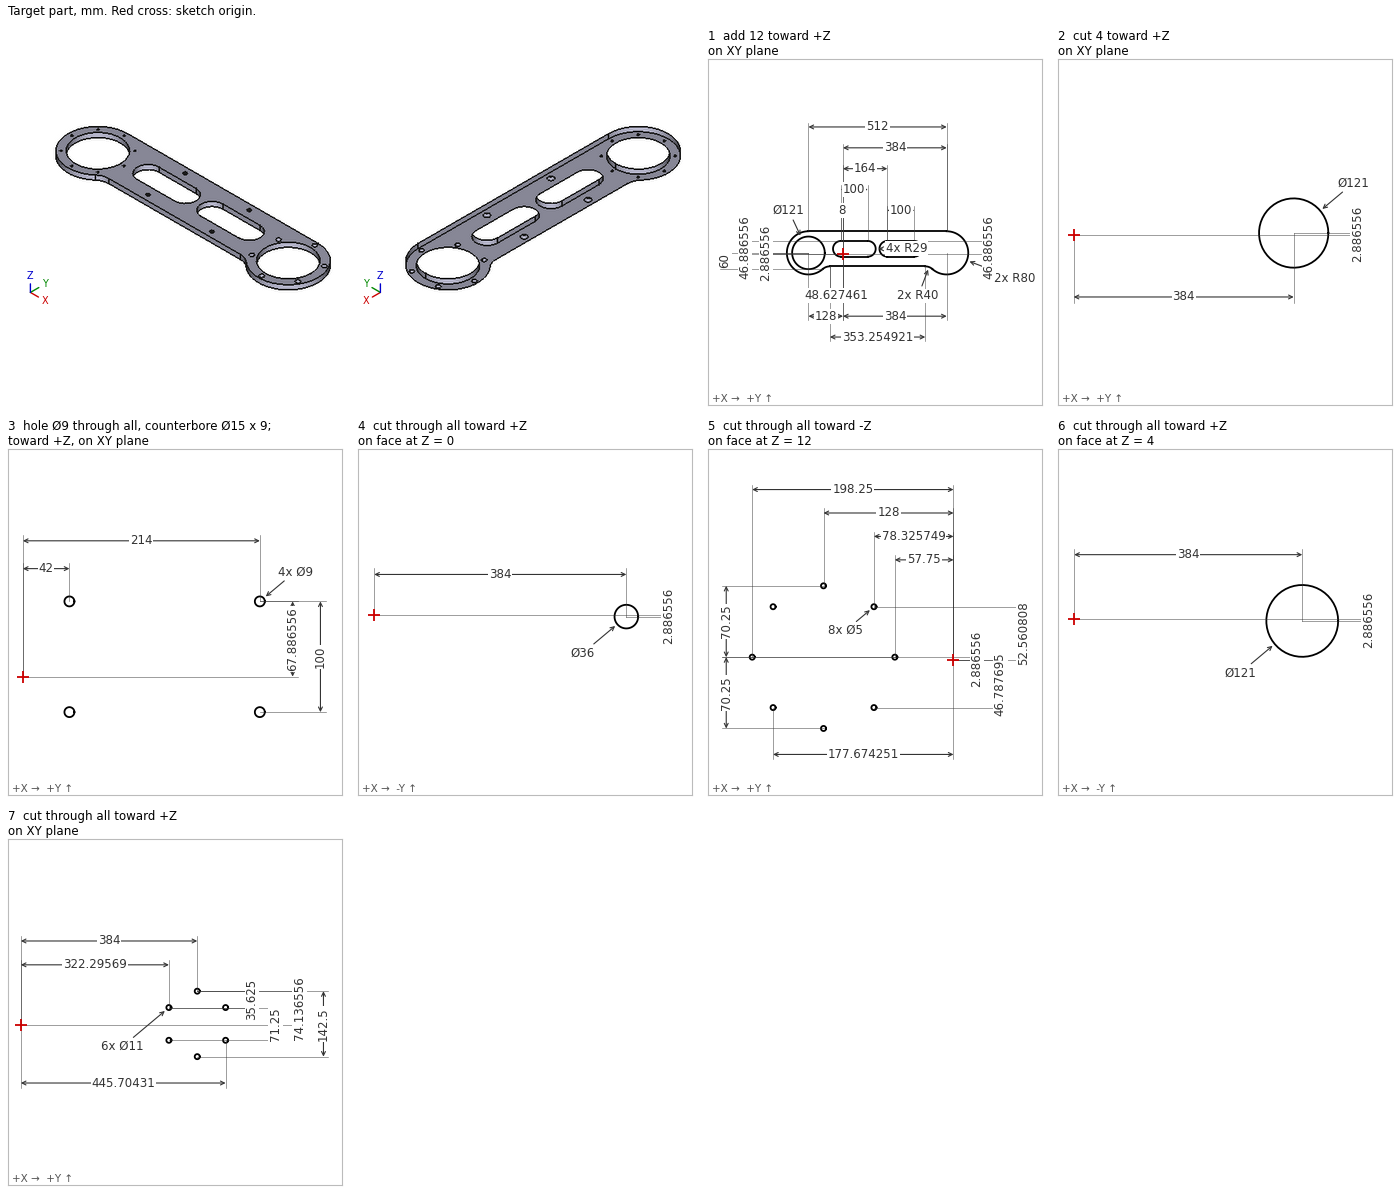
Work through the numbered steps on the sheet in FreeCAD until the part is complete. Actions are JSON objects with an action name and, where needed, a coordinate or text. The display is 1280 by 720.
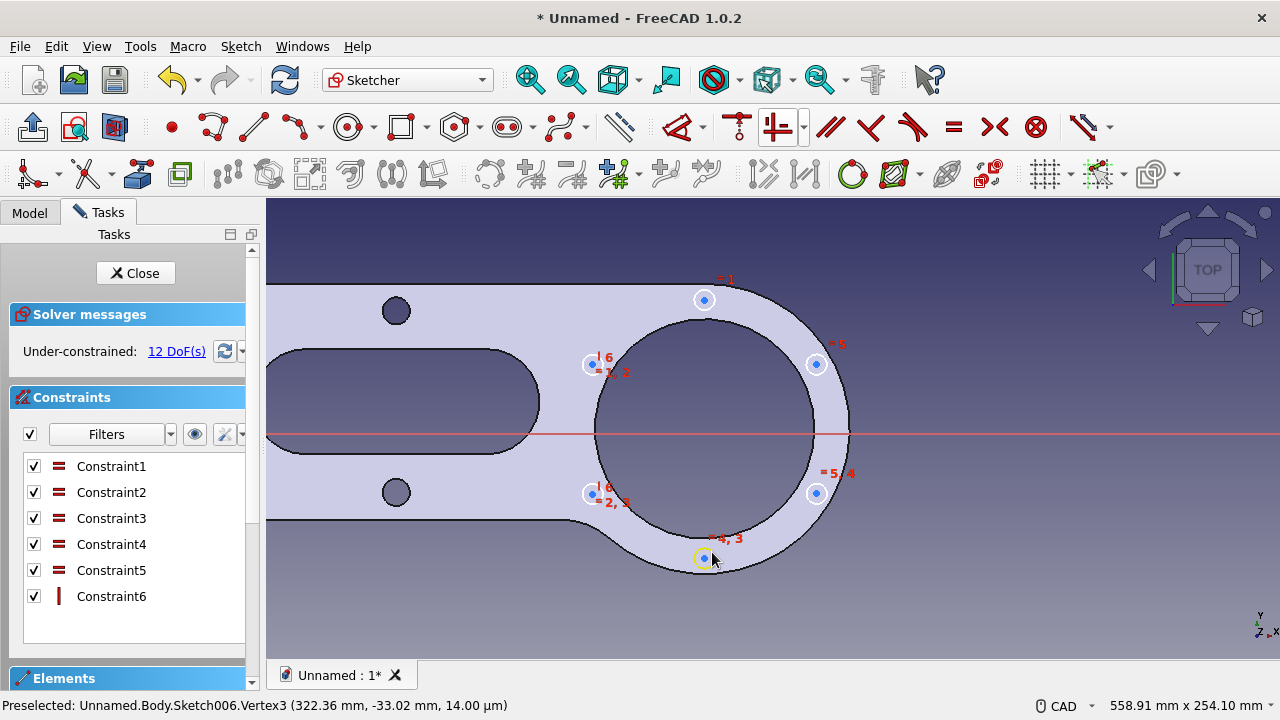
{"action": "left_click", "coordinate": [705, 300]}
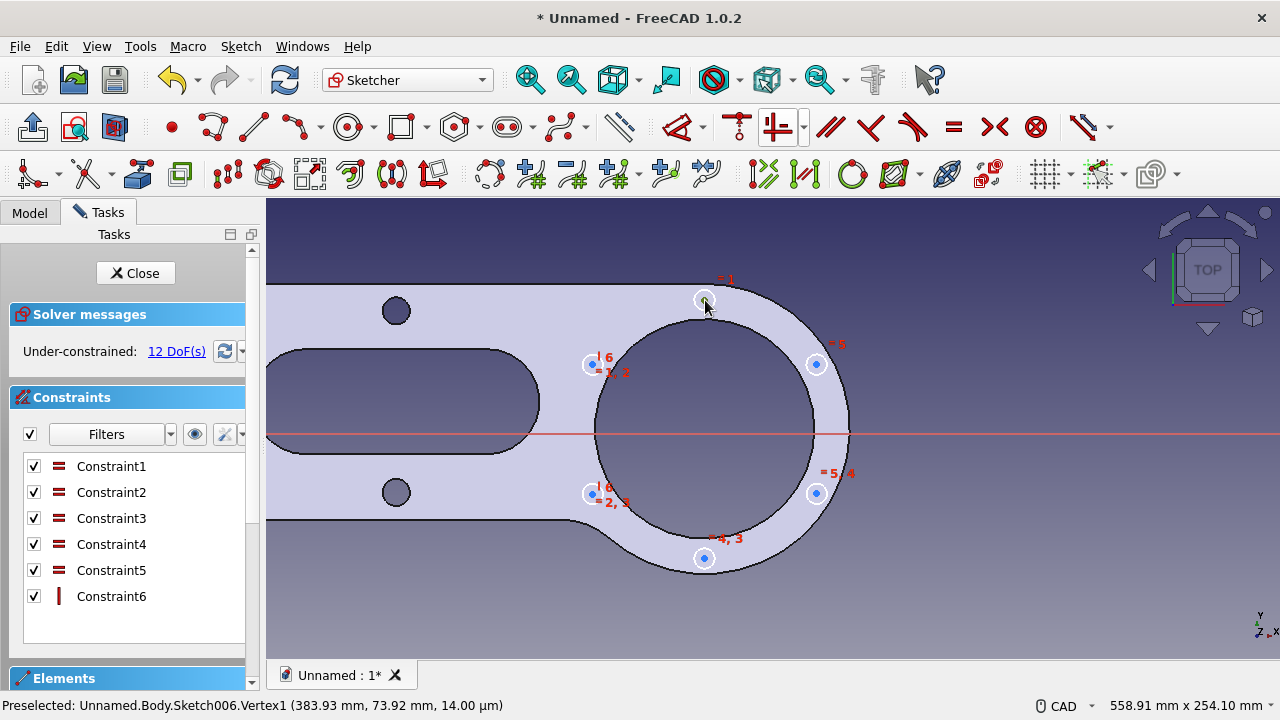
{"action": "left_click", "coordinate": [705, 558]}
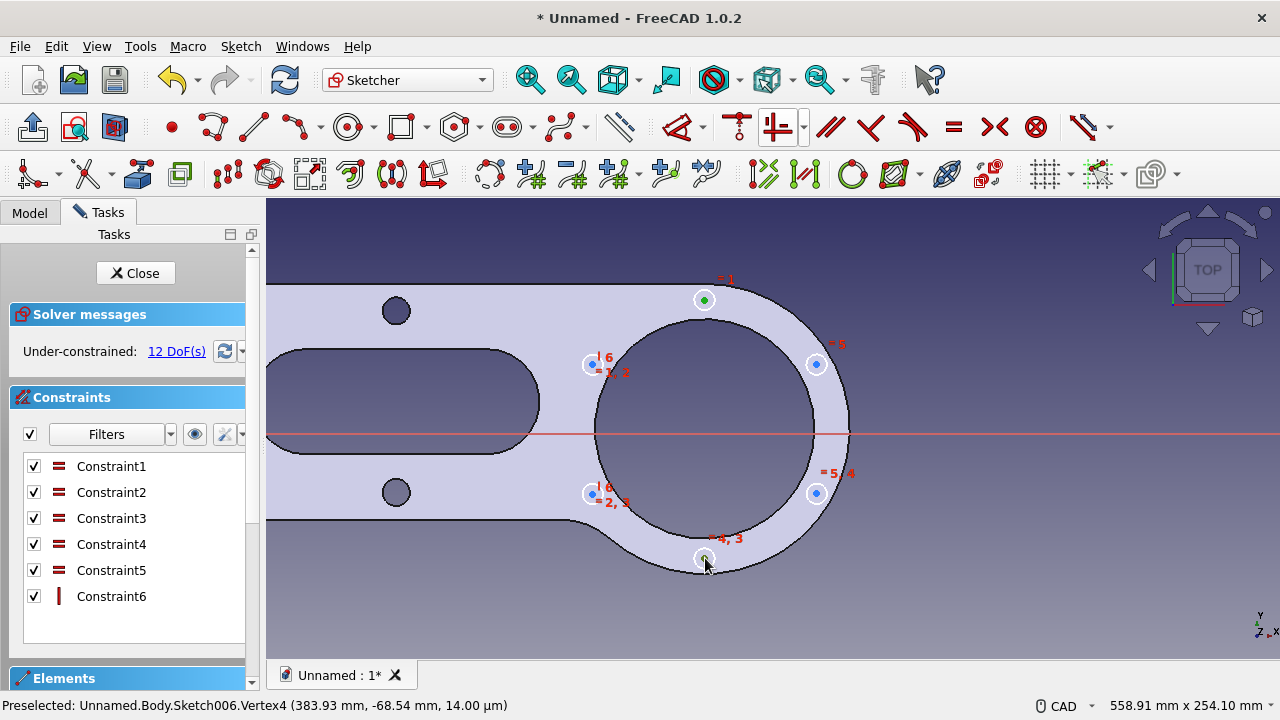
{"action": "left_click", "coordinate": [804, 128]}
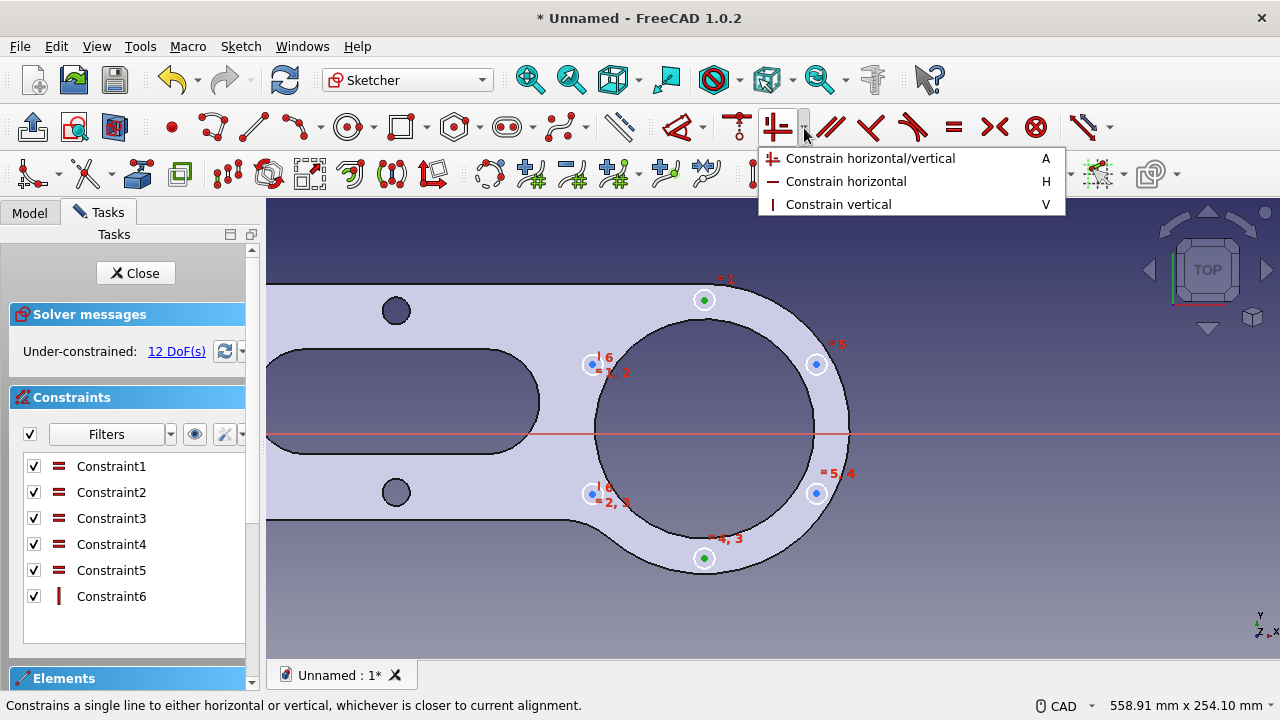
{"action": "left_click", "coordinate": [912, 204]}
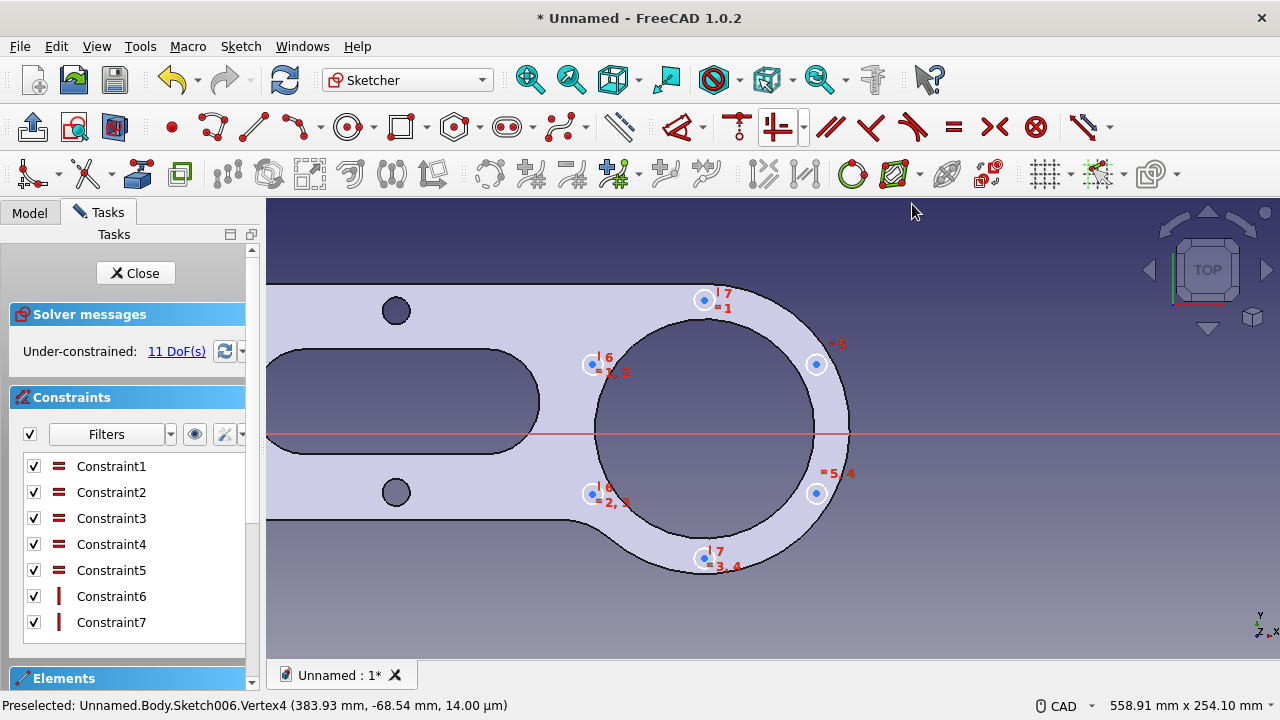
{"action": "left_click", "coordinate": [591, 496]}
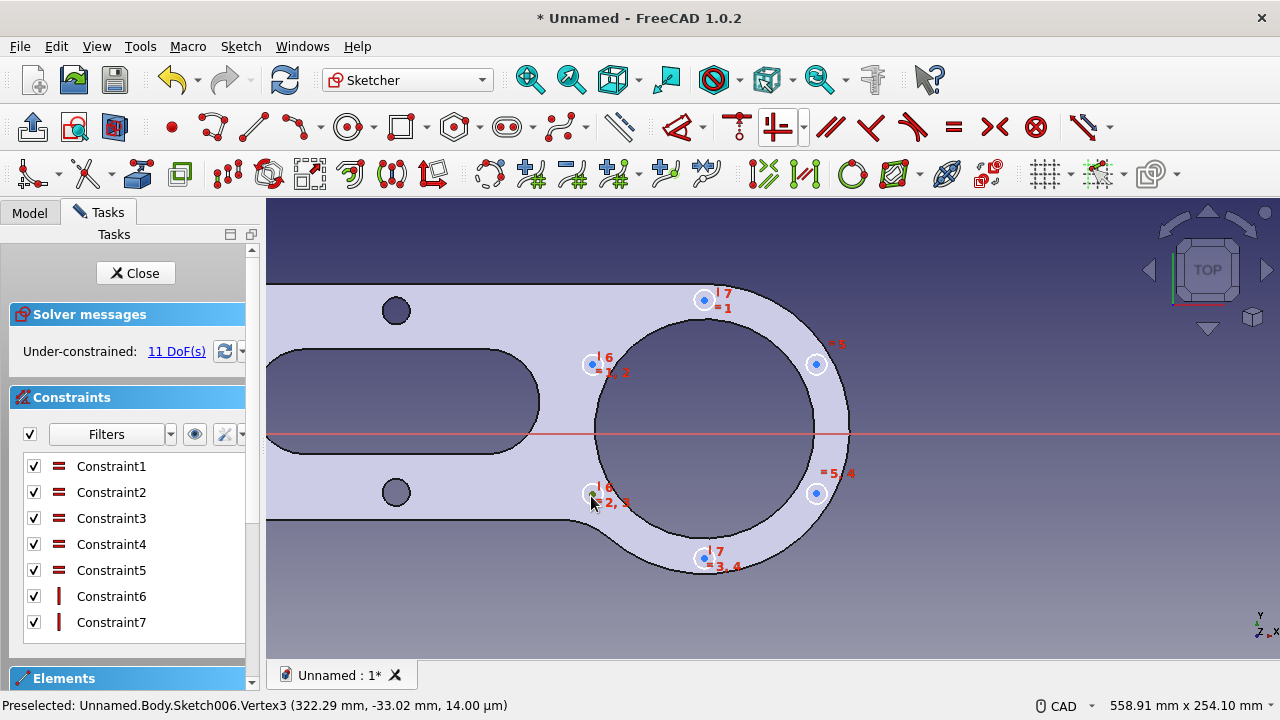
{"action": "left_click", "coordinate": [817, 494]}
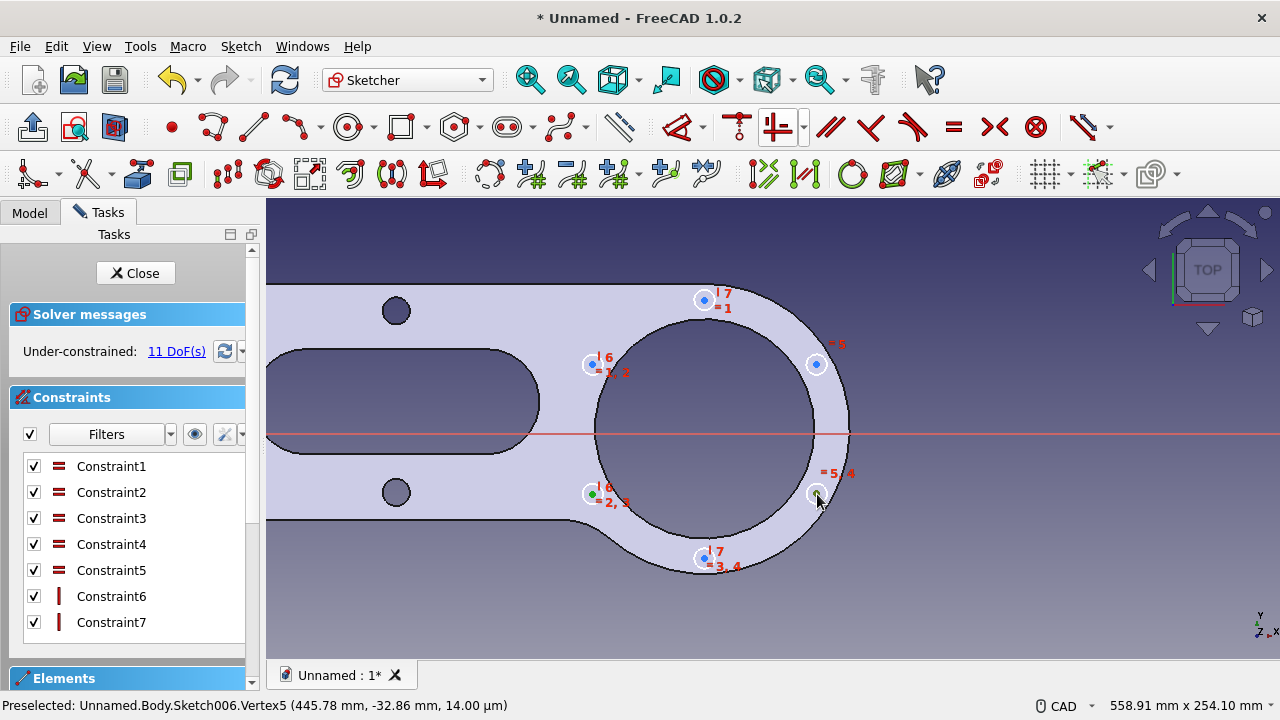
{"action": "left_click", "coordinate": [804, 128]}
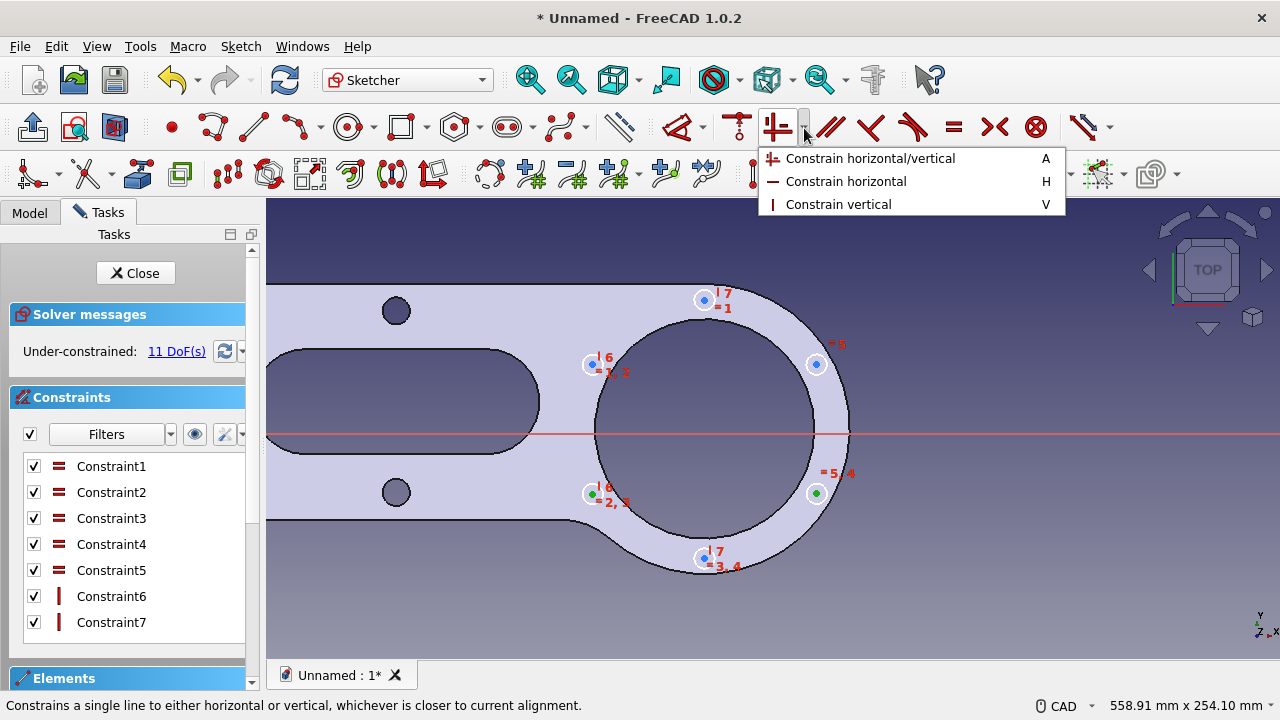
{"action": "left_click", "coordinate": [912, 182]}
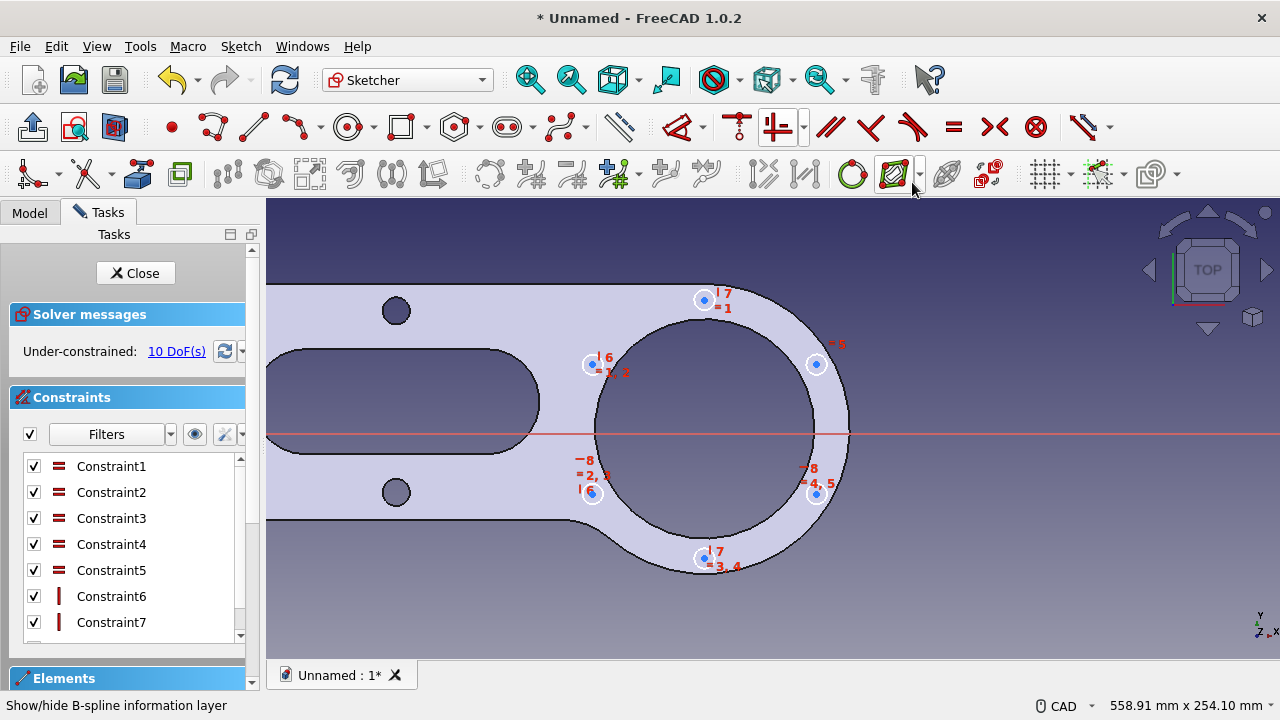
{"action": "left_click", "coordinate": [817, 494]}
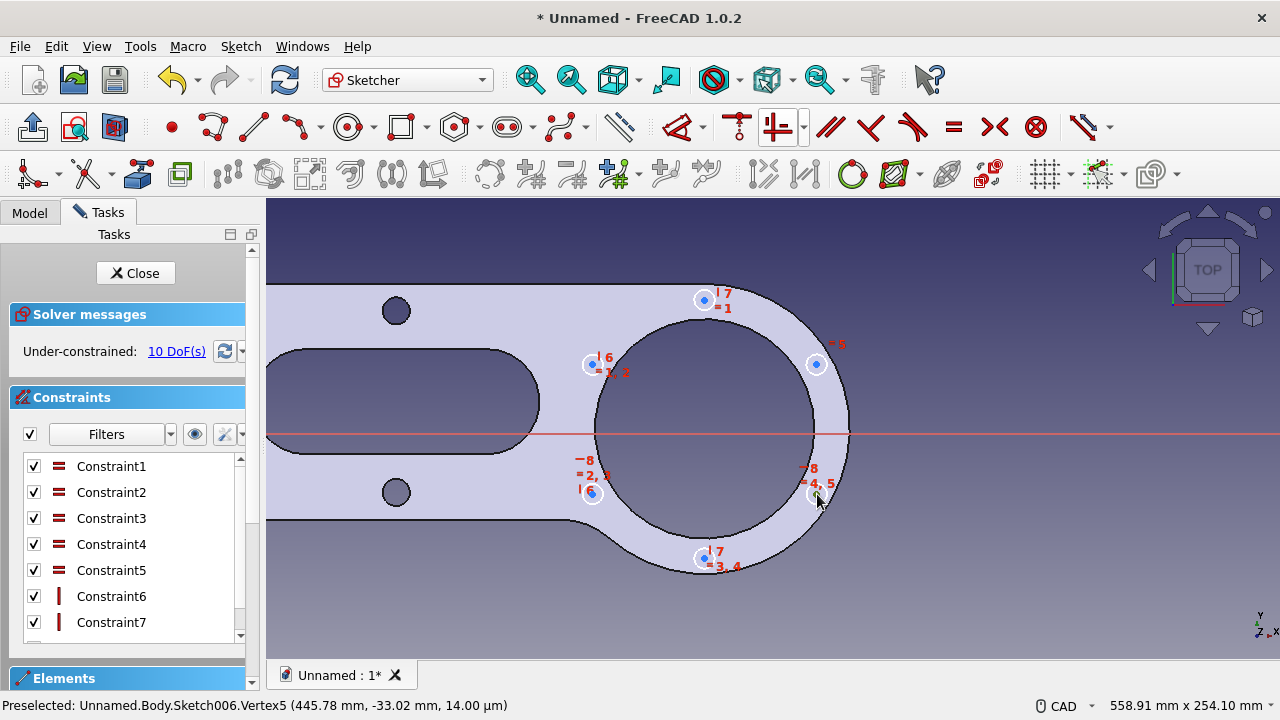
{"action": "left_click", "coordinate": [817, 365]}